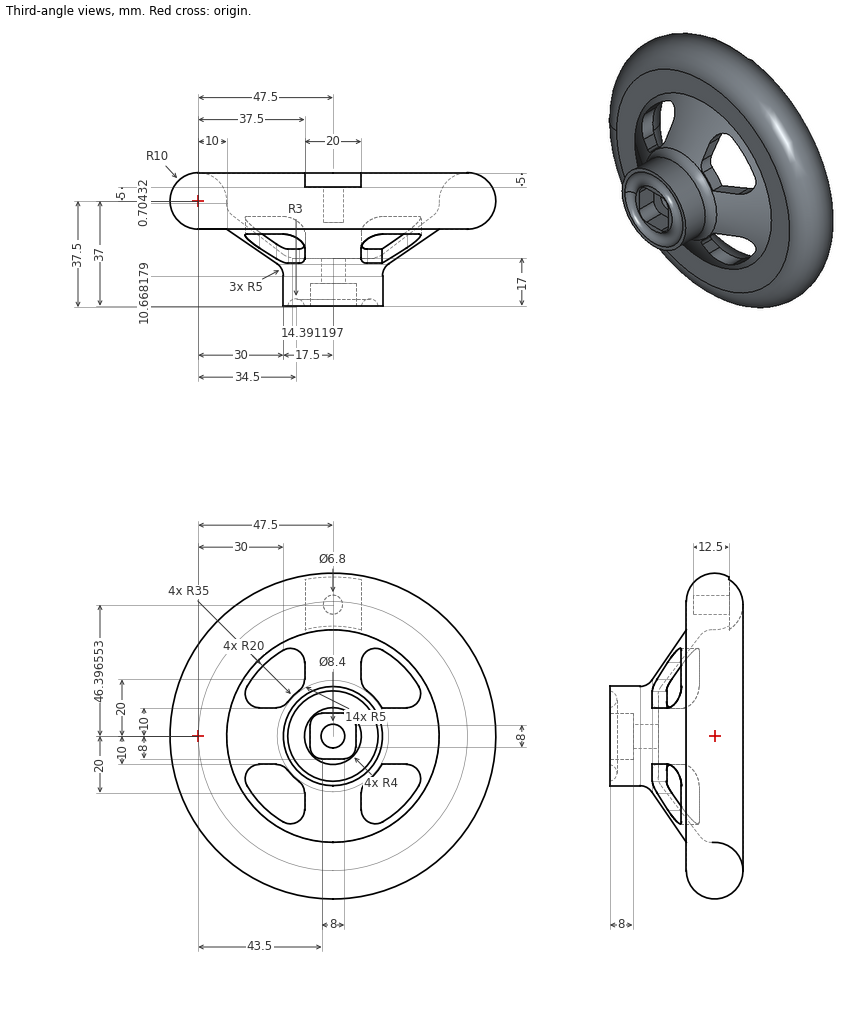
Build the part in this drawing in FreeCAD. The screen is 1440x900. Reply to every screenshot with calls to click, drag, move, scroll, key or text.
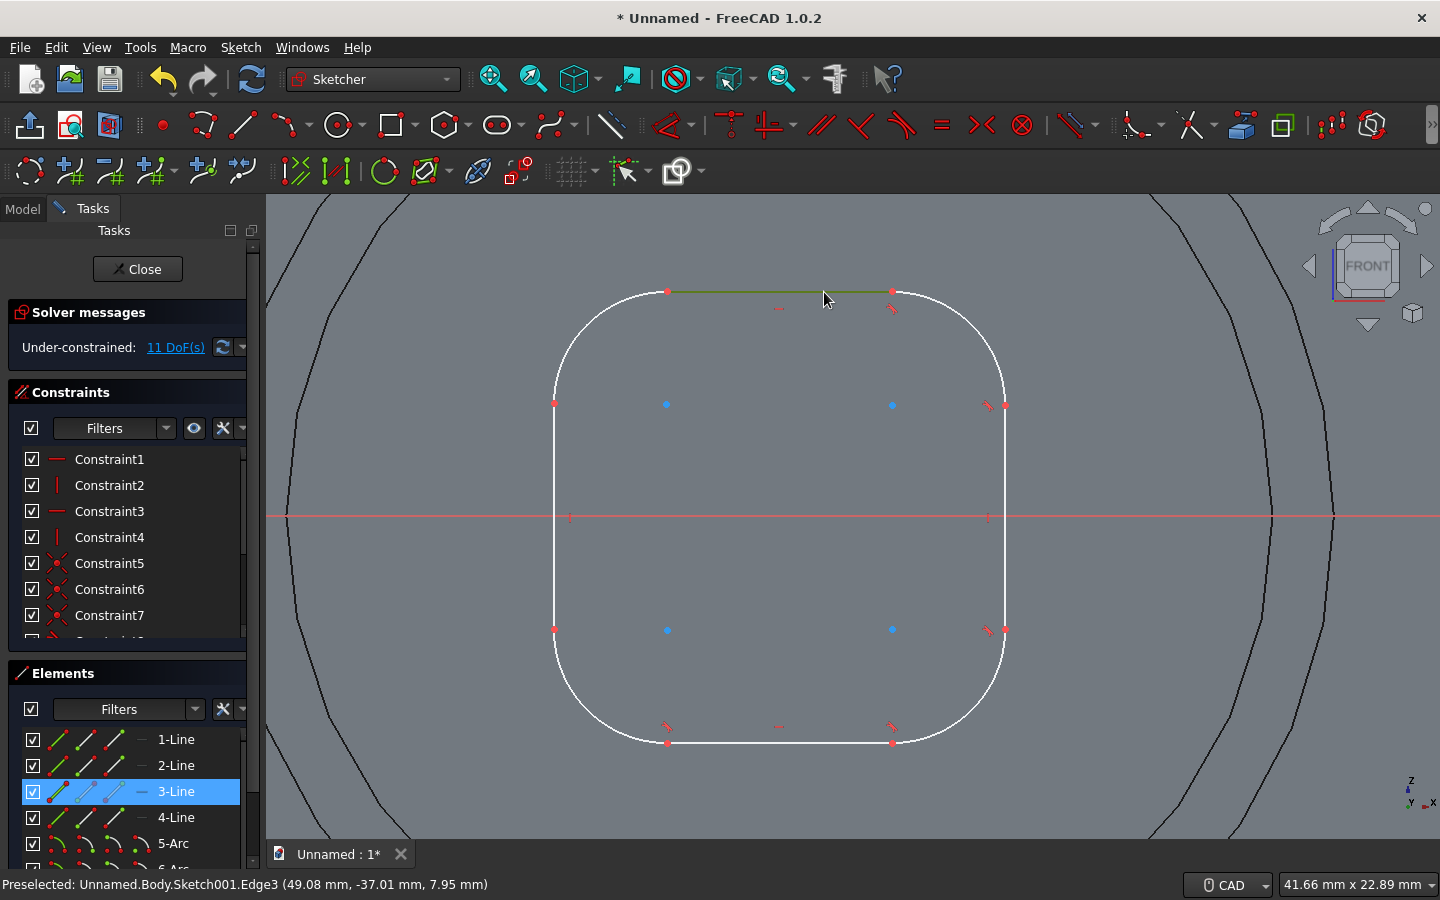
click(616, 304)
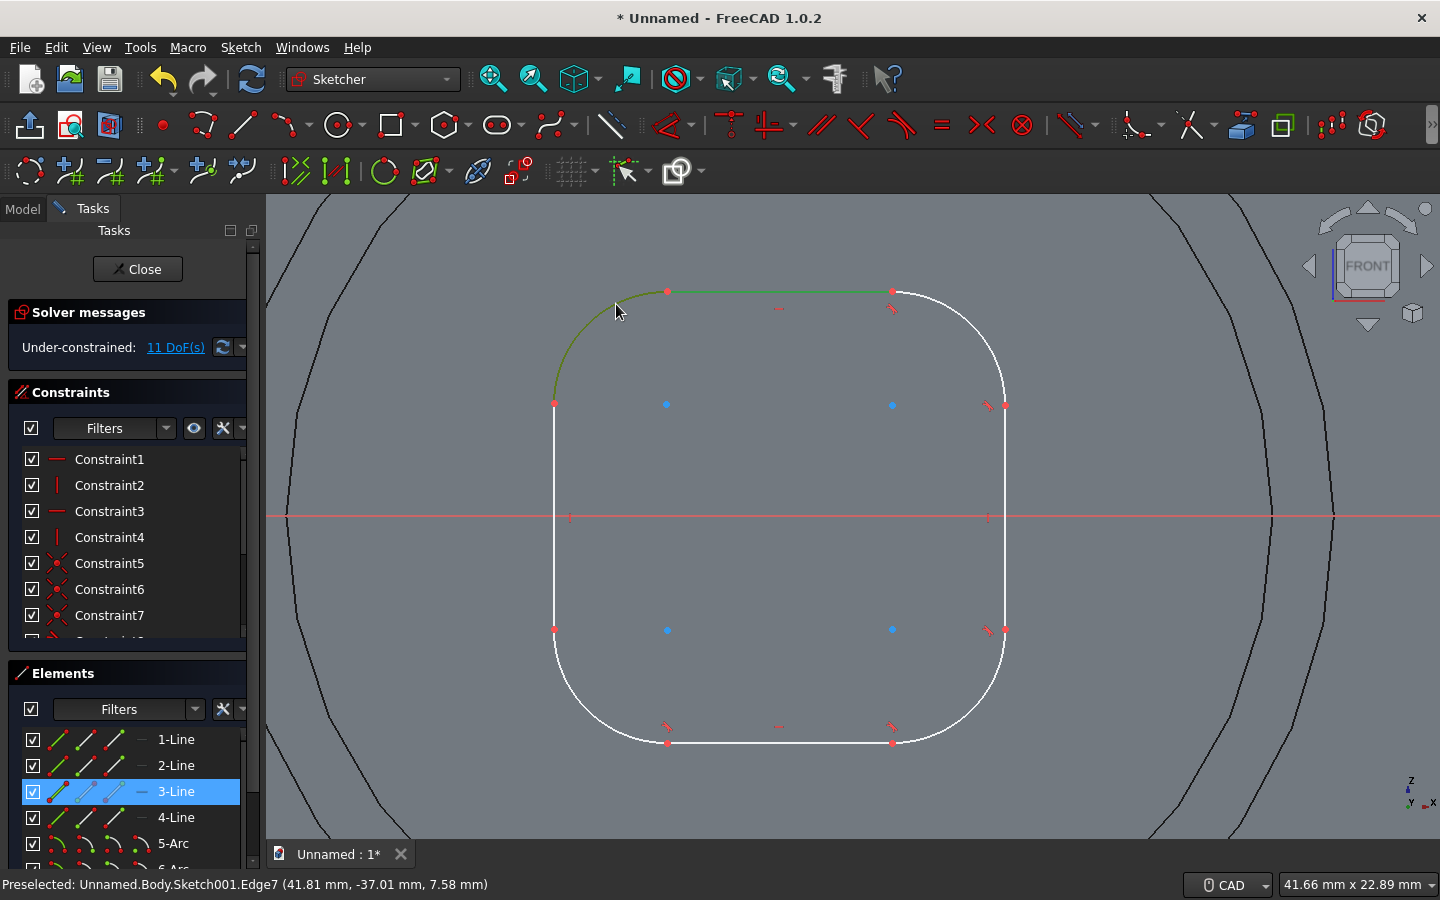
click(902, 126)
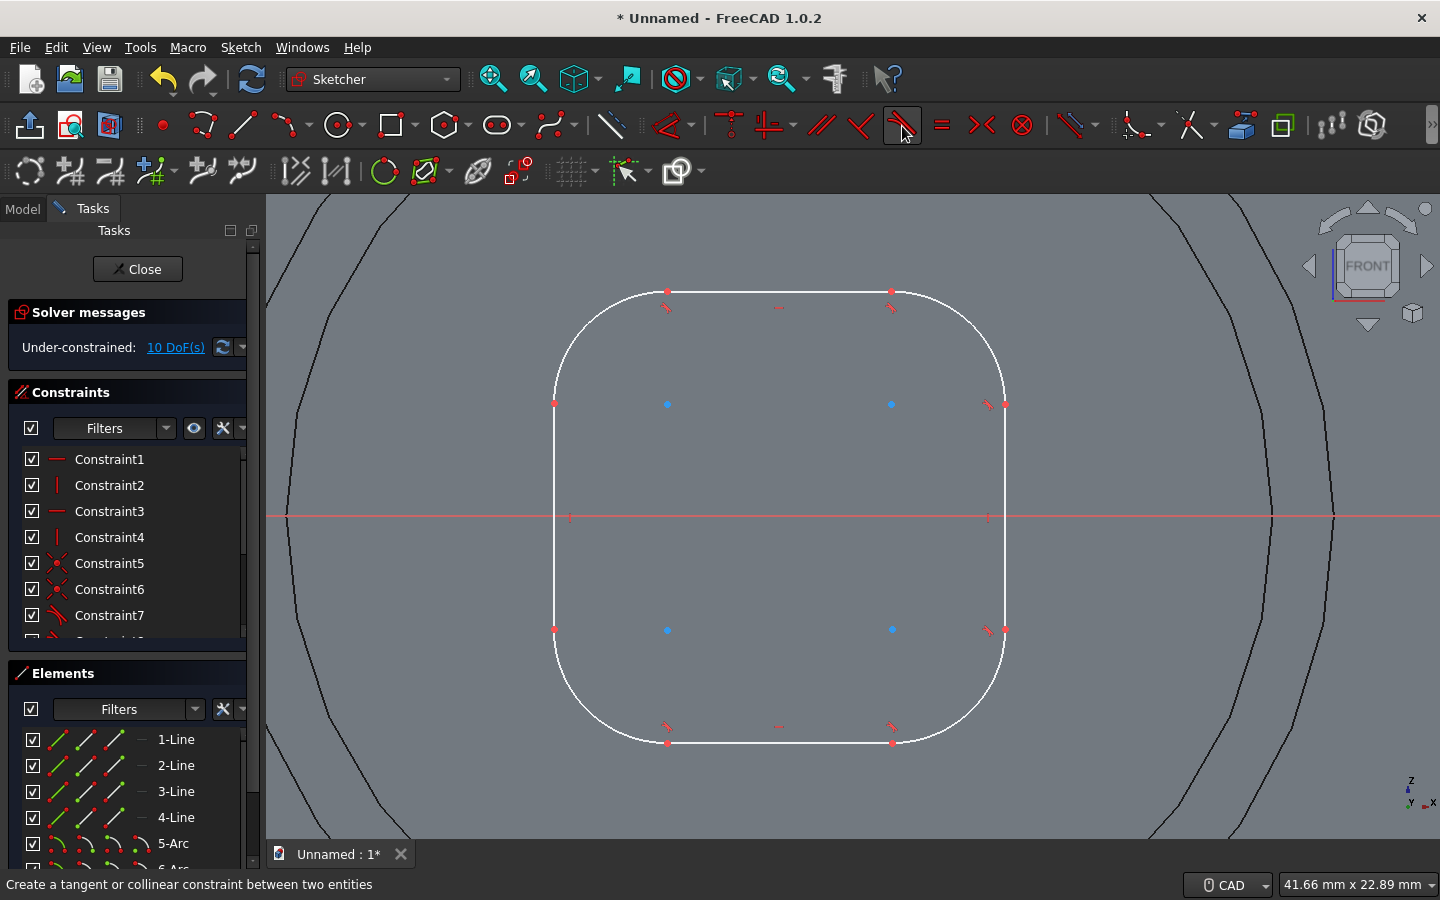
click(554, 472)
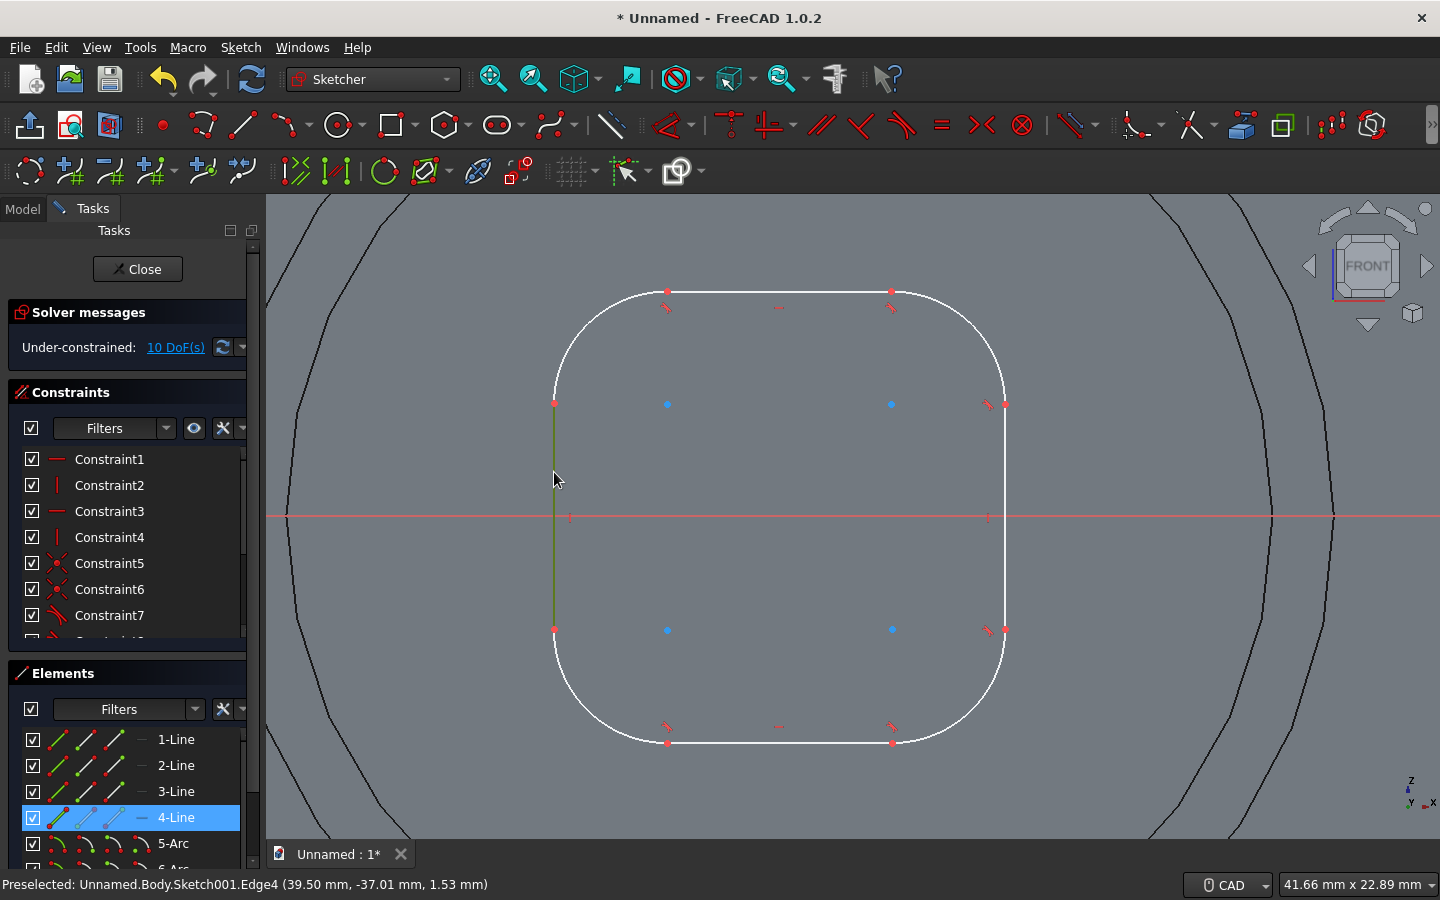
click(616, 304)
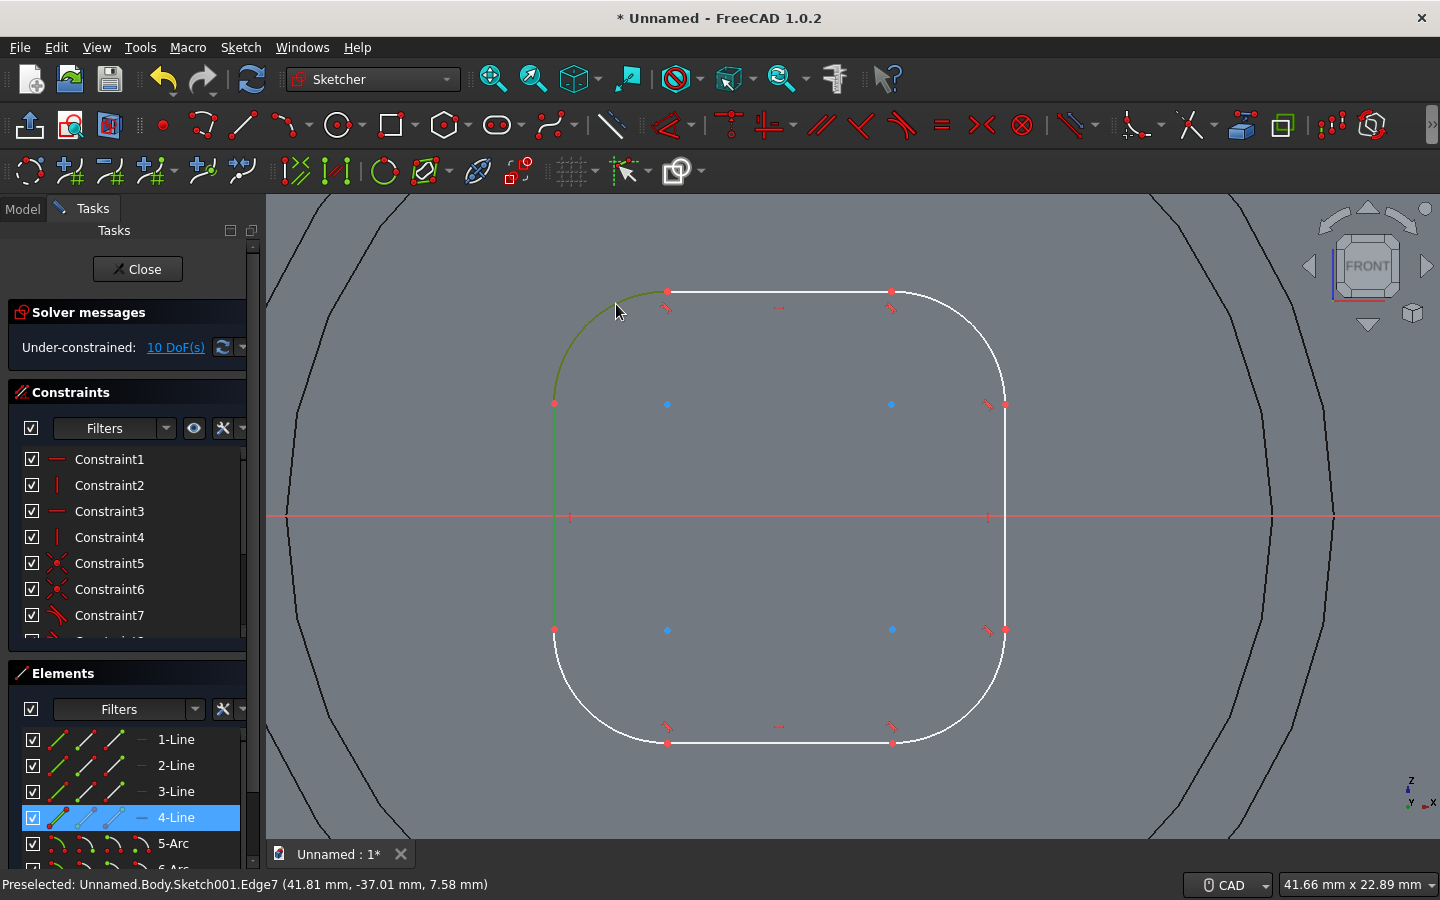
click(902, 126)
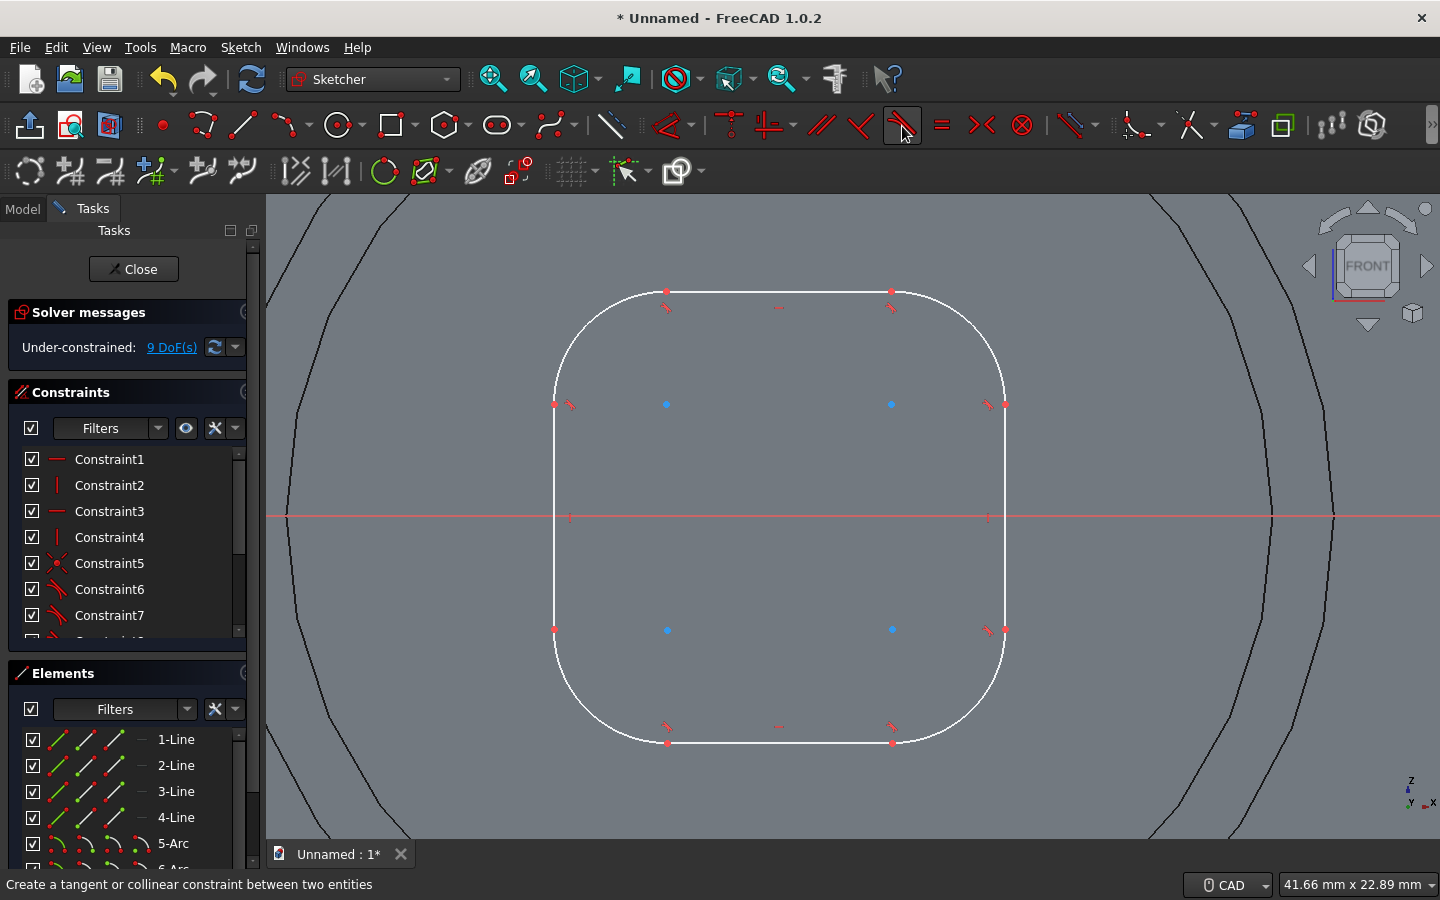
click(554, 472)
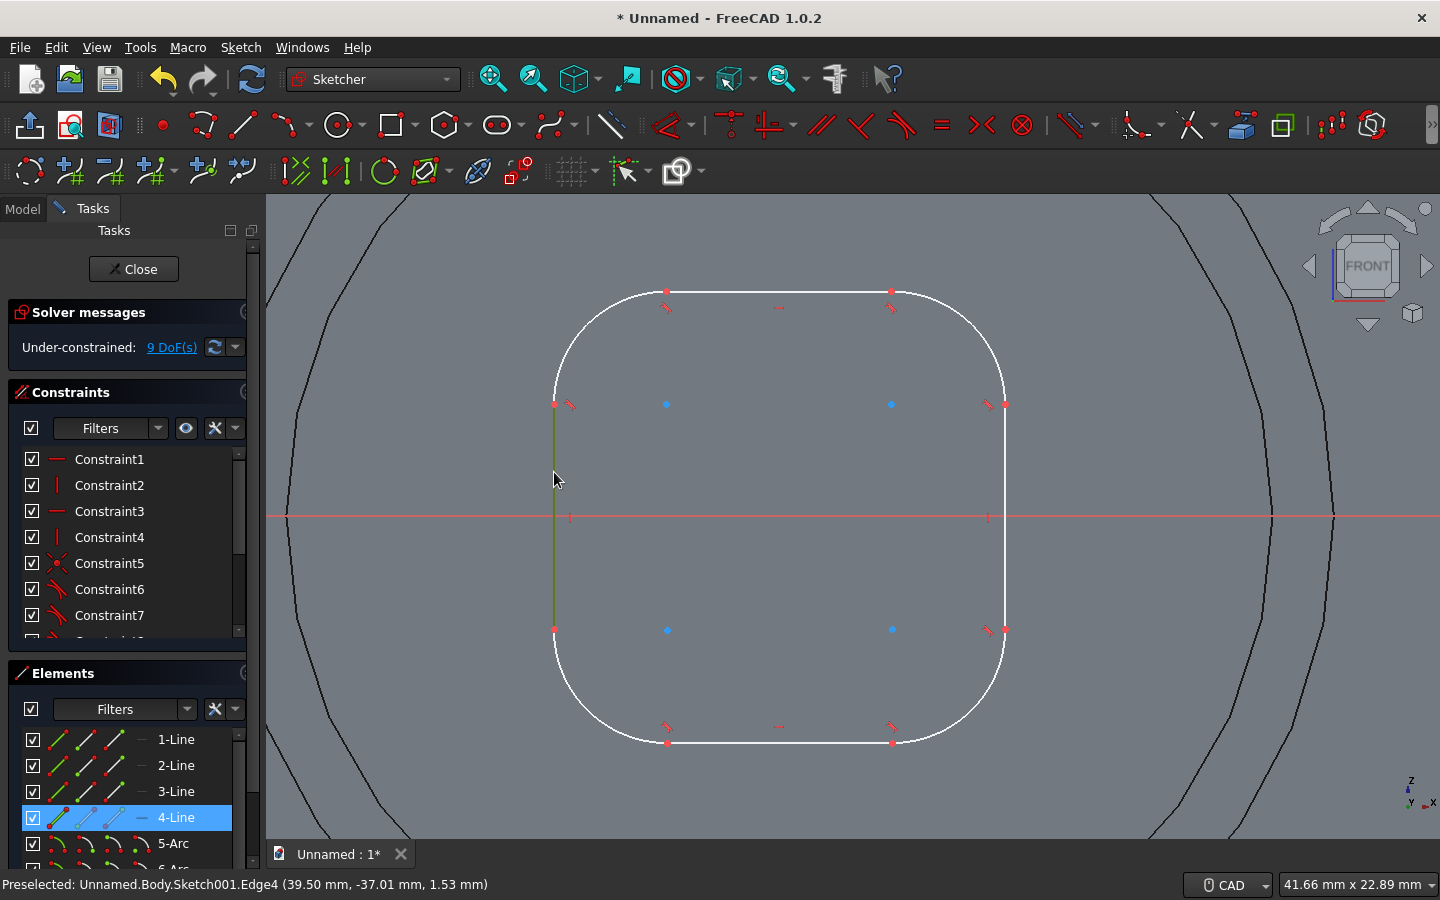
click(566, 681)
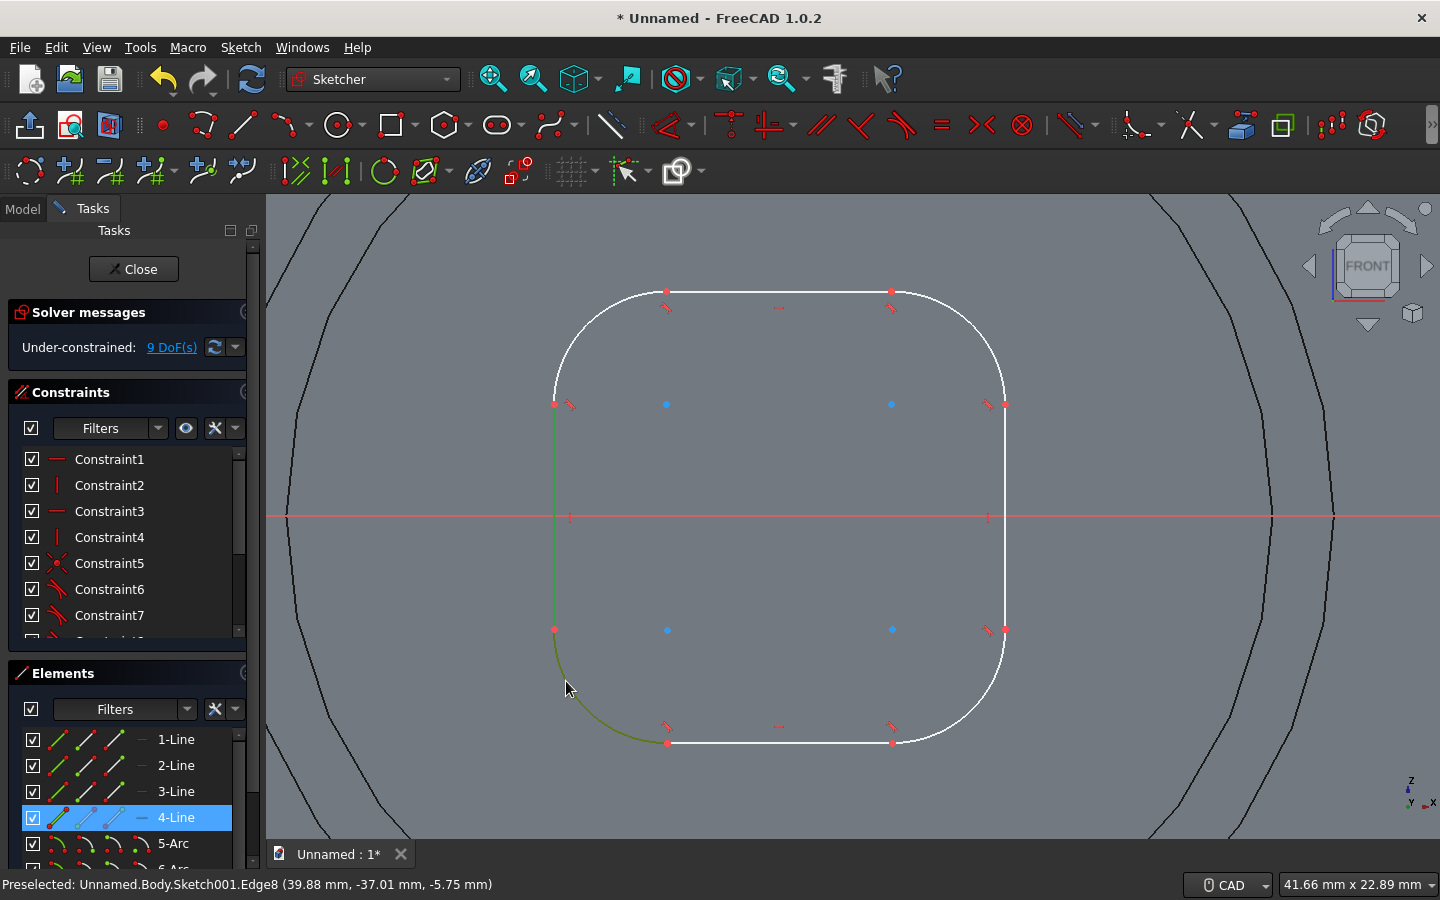
click(902, 126)